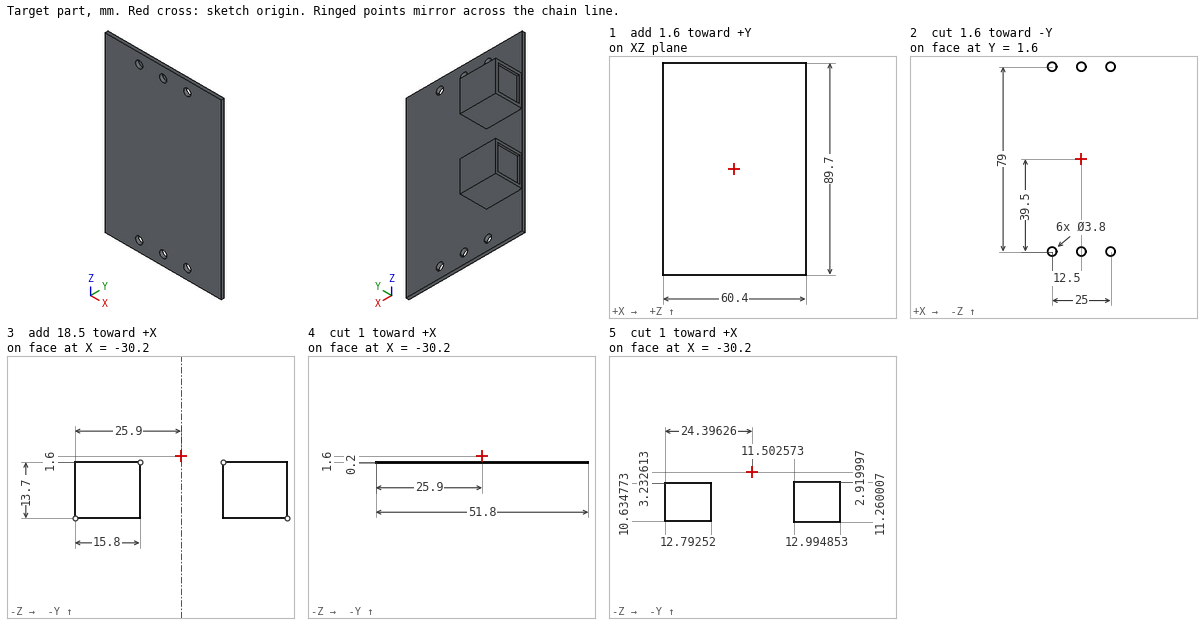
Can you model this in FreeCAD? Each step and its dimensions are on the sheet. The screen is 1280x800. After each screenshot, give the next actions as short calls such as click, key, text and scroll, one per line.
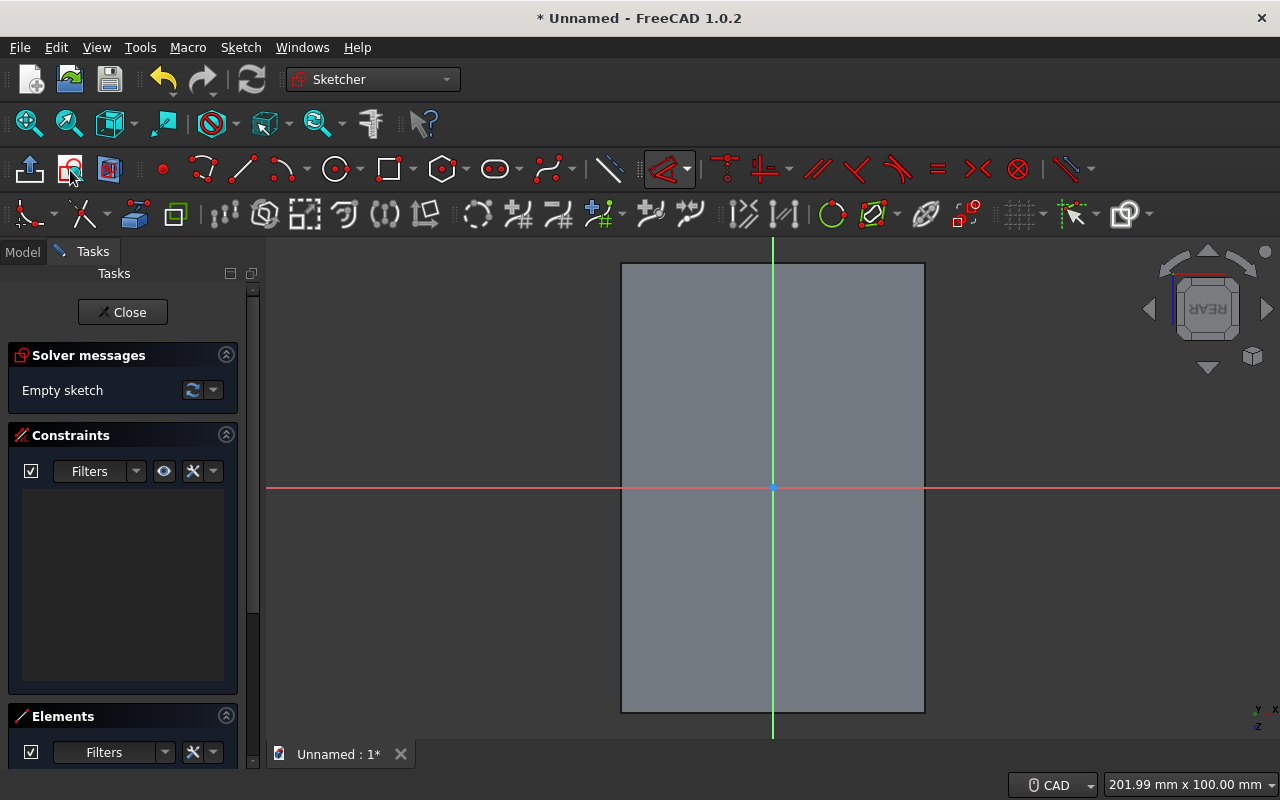
scroll(395, 488, down, 1)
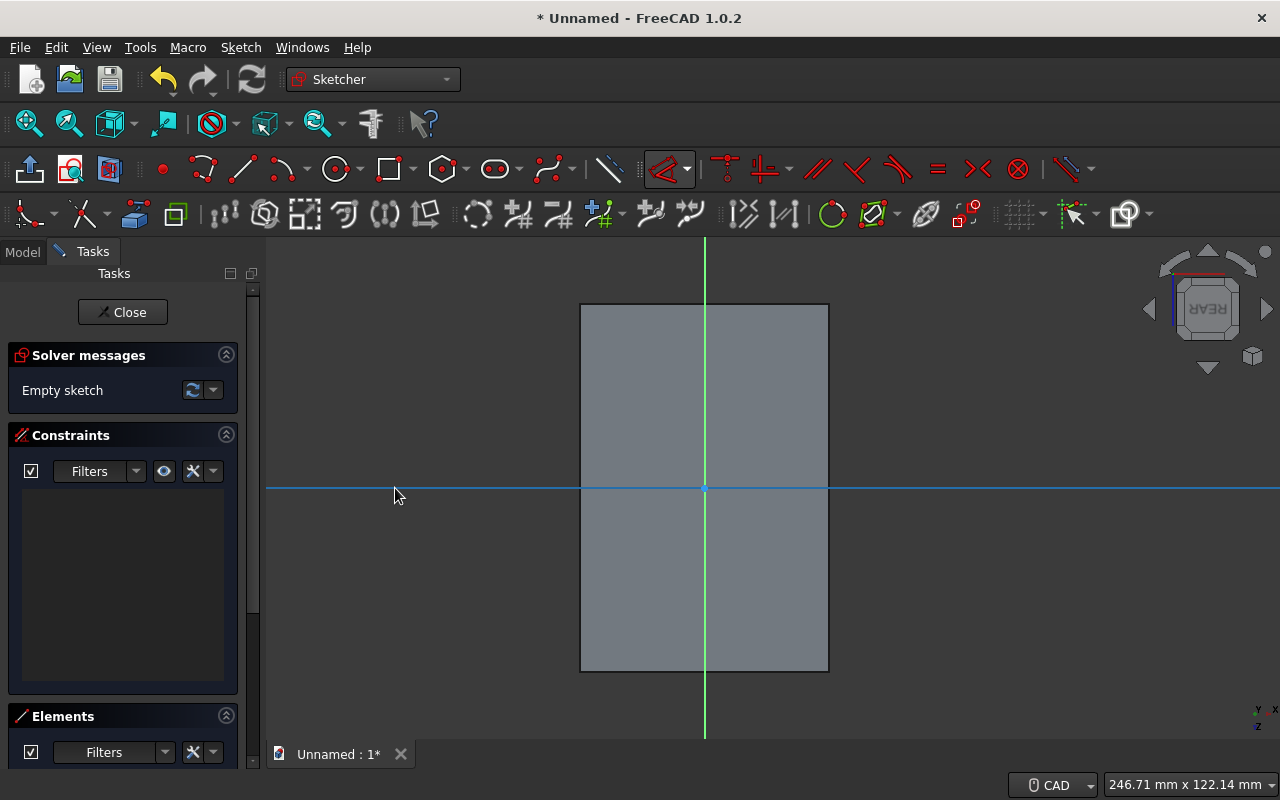
click(336, 170)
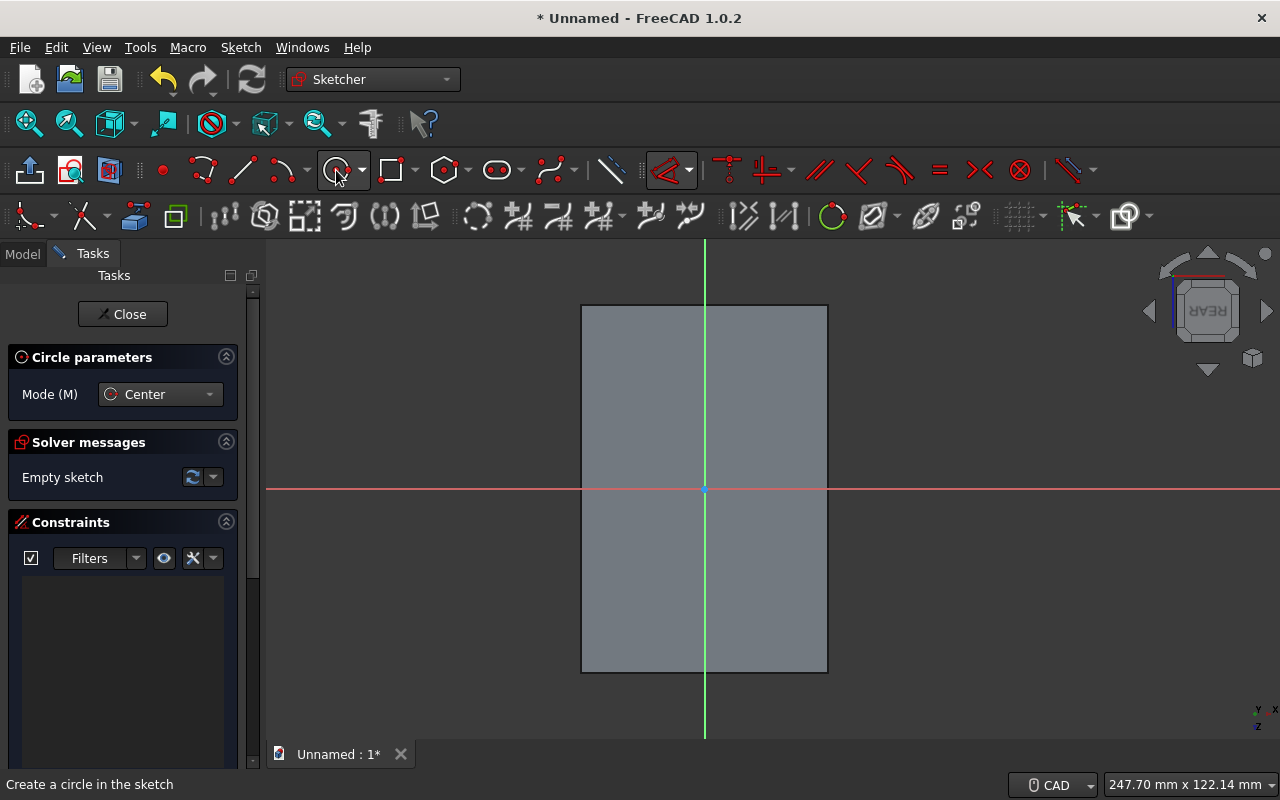
scroll(654, 651, up, 6)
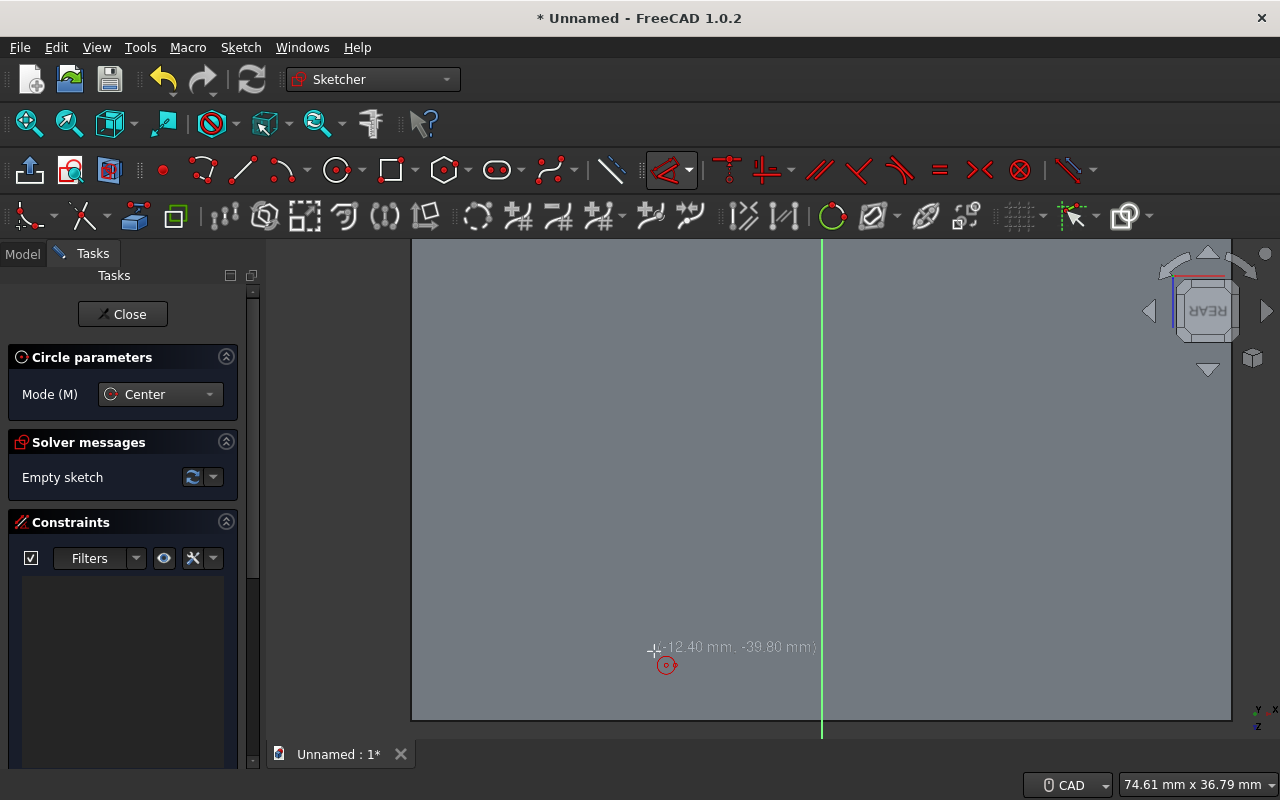
click(652, 648)
click(670, 630)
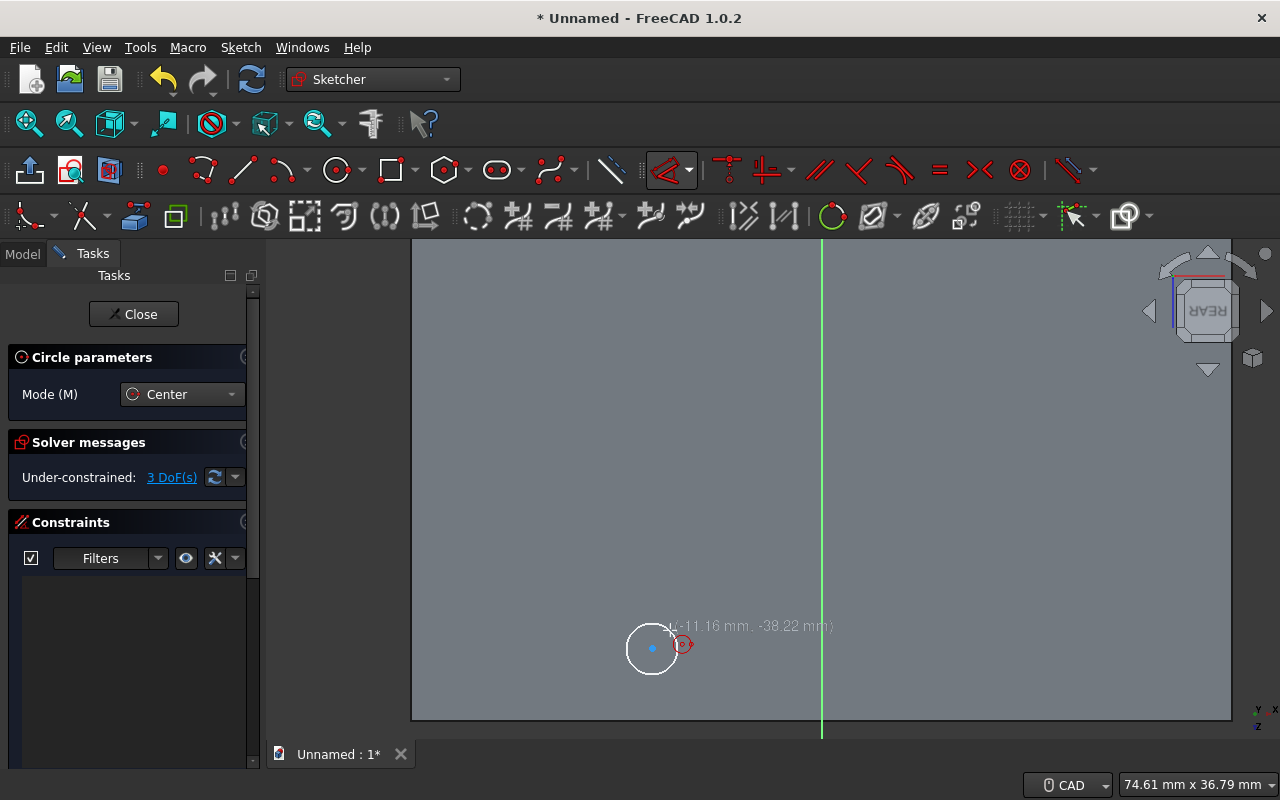
click(992, 648)
click(1010, 630)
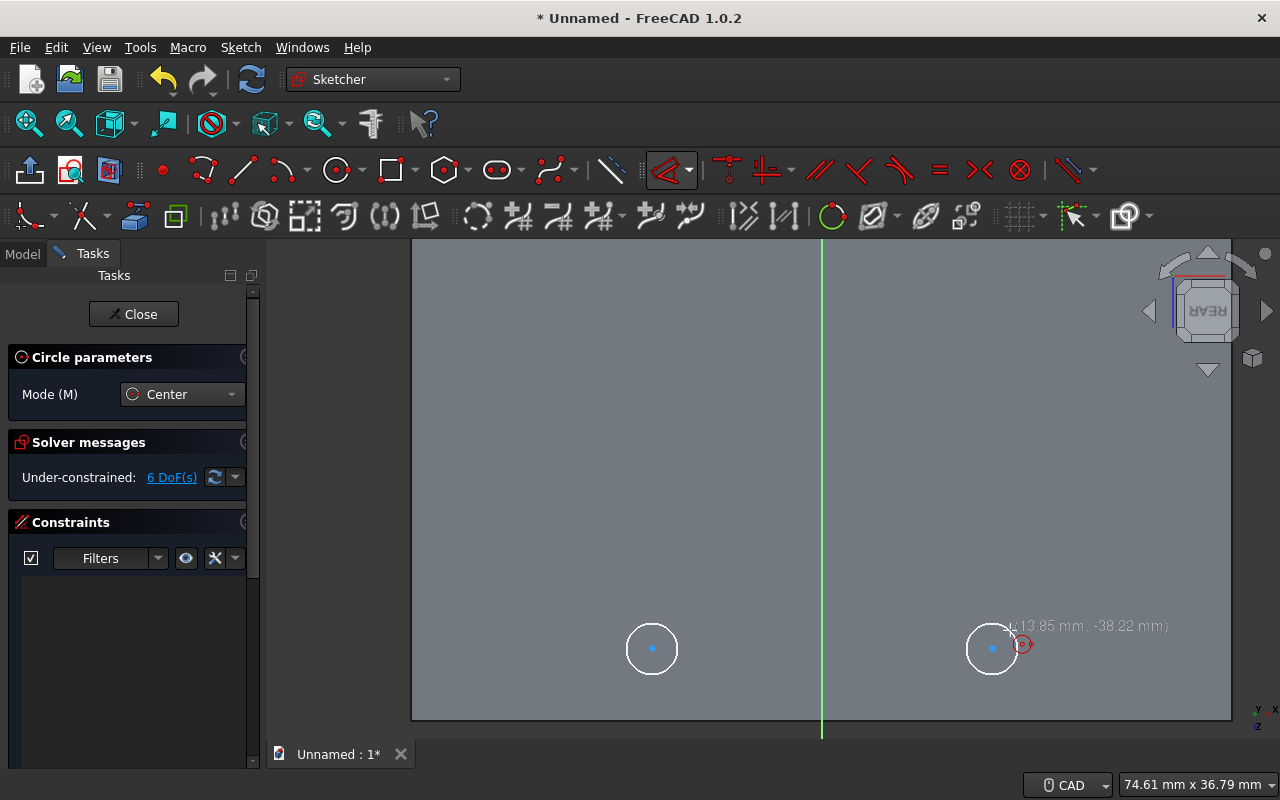
scroll(654, 652, down, 6)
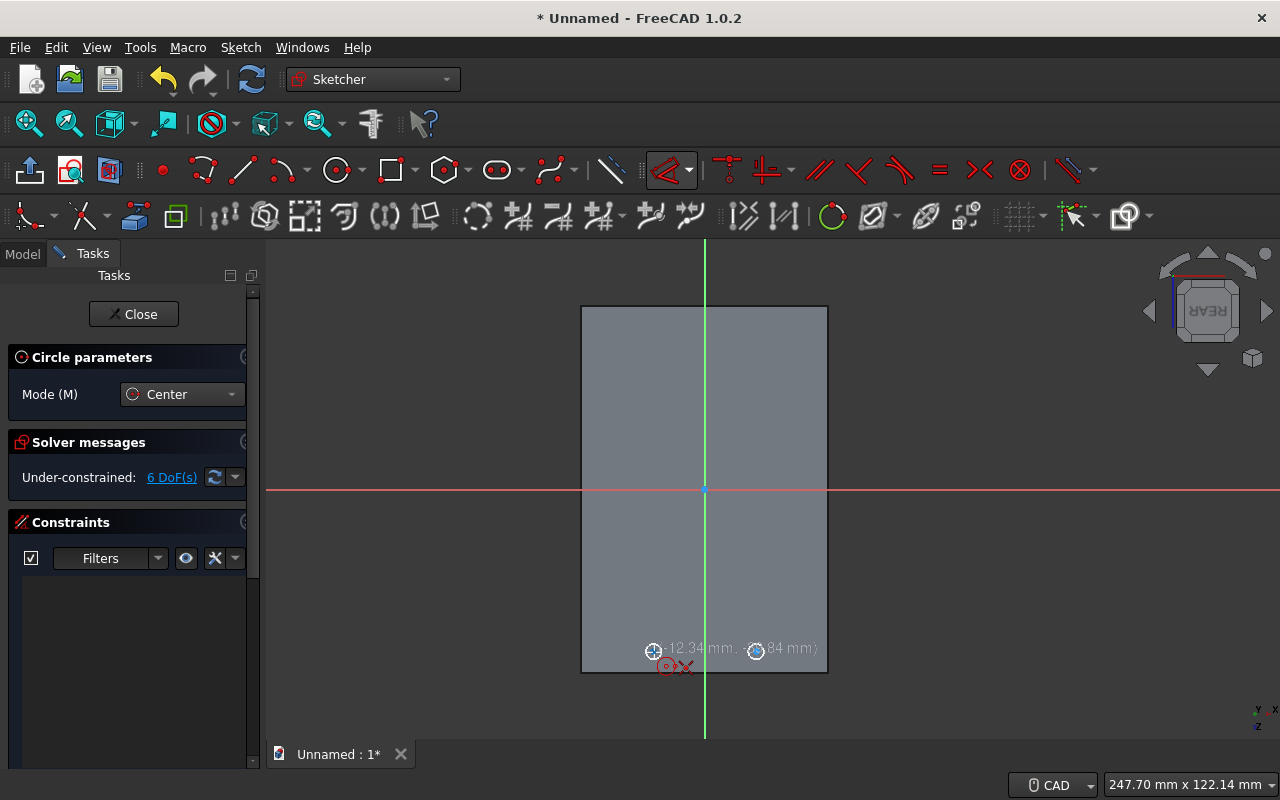
scroll(654, 328, up, 6)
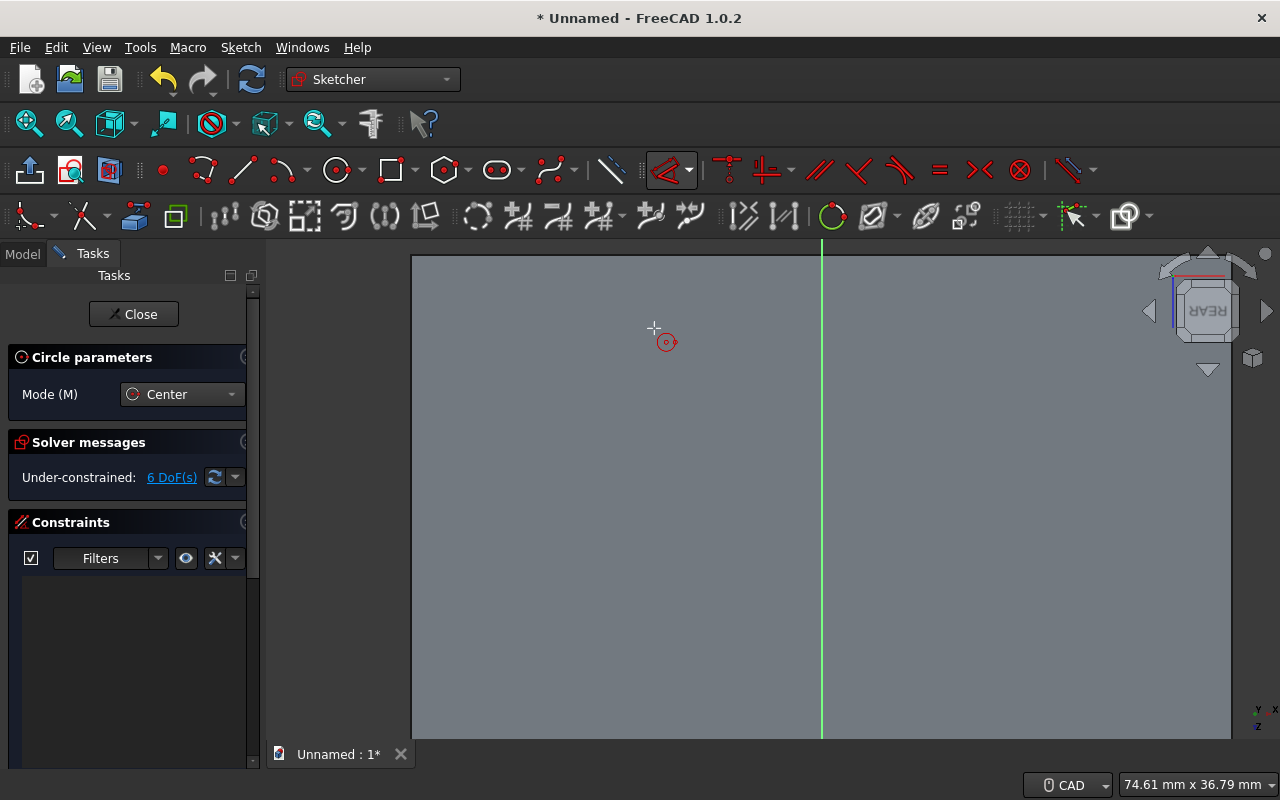
click(652, 328)
click(670, 310)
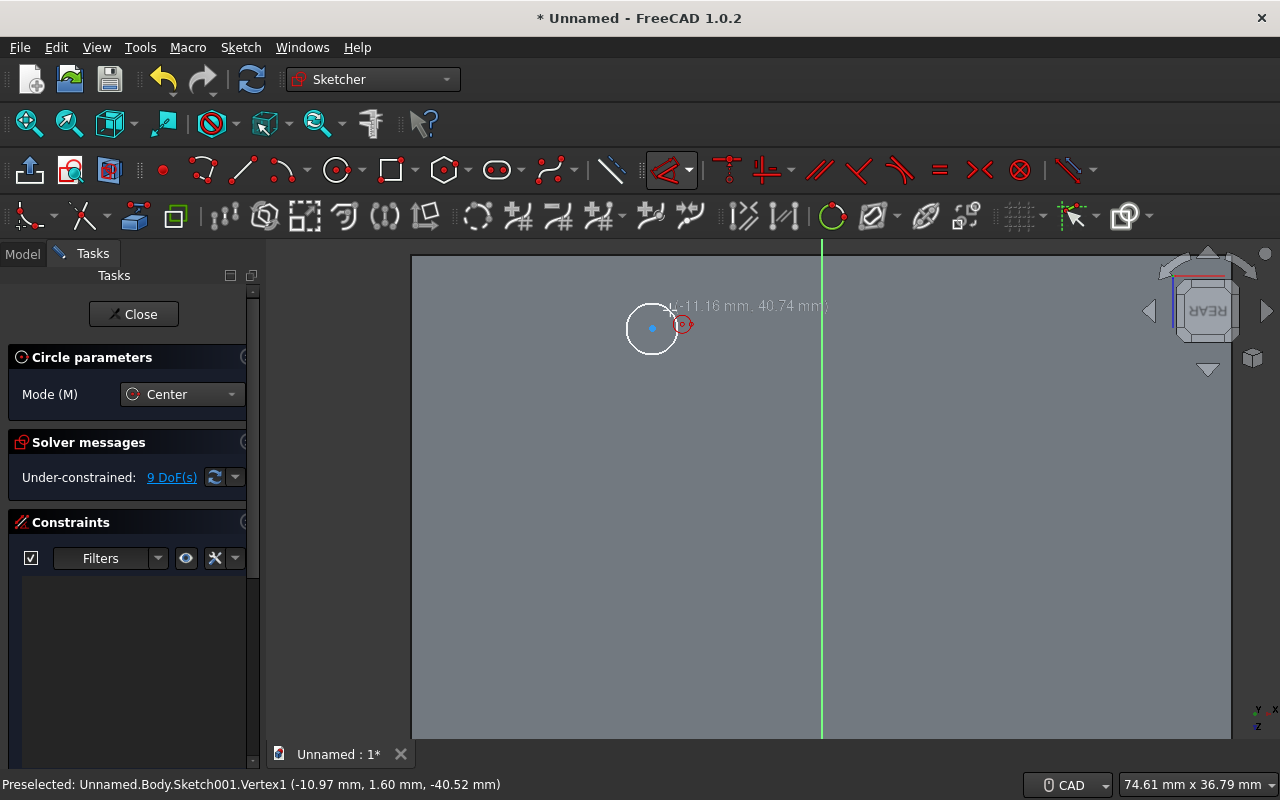
click(992, 328)
click(1010, 310)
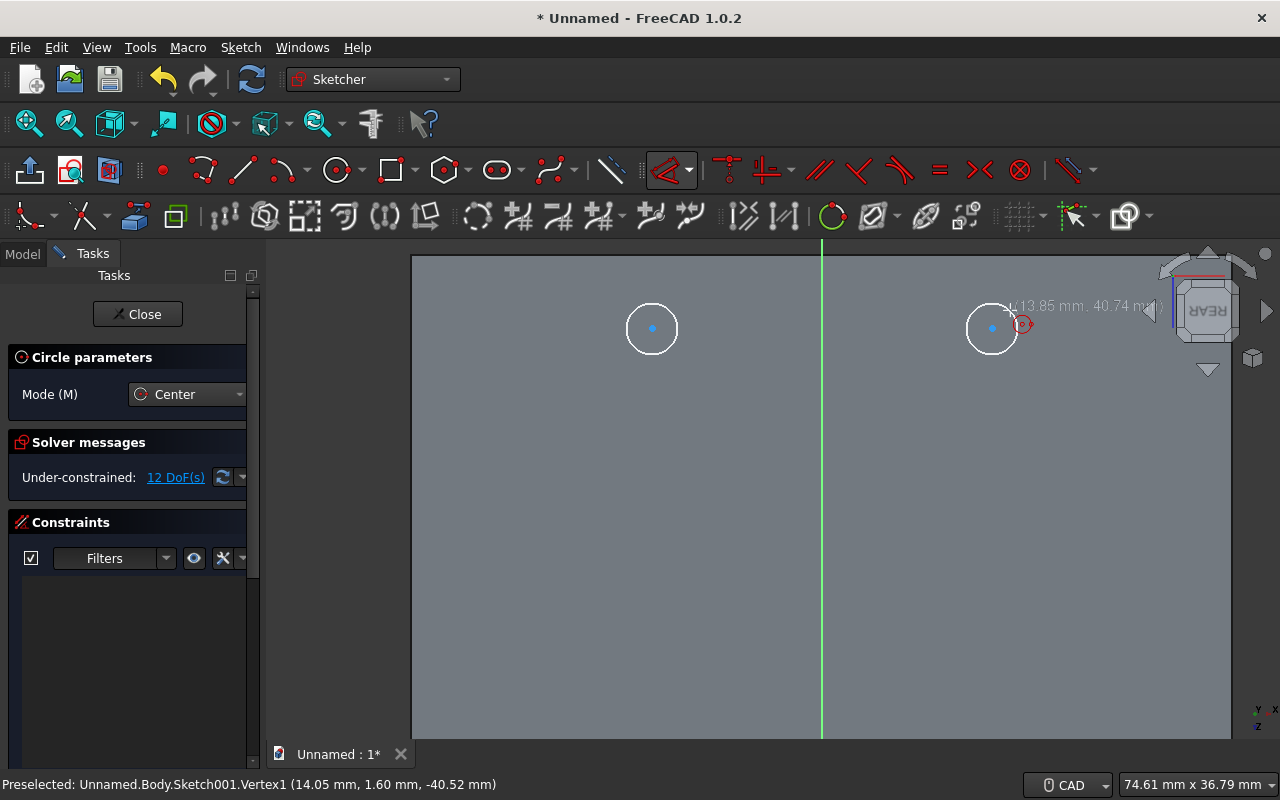
click(822, 328)
click(840, 310)